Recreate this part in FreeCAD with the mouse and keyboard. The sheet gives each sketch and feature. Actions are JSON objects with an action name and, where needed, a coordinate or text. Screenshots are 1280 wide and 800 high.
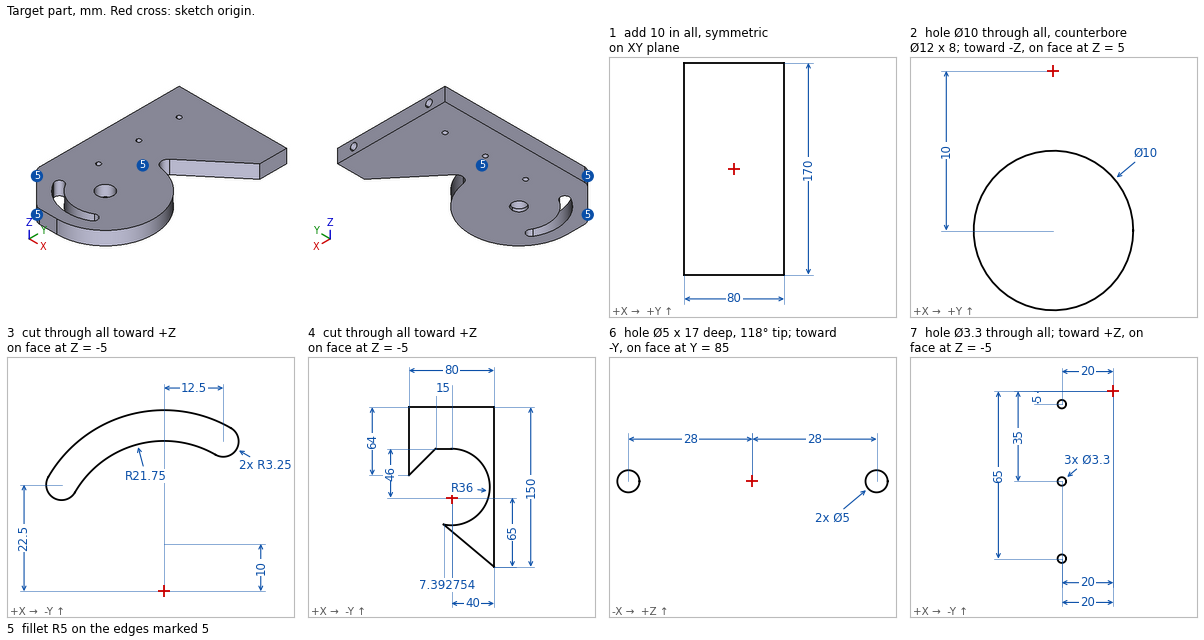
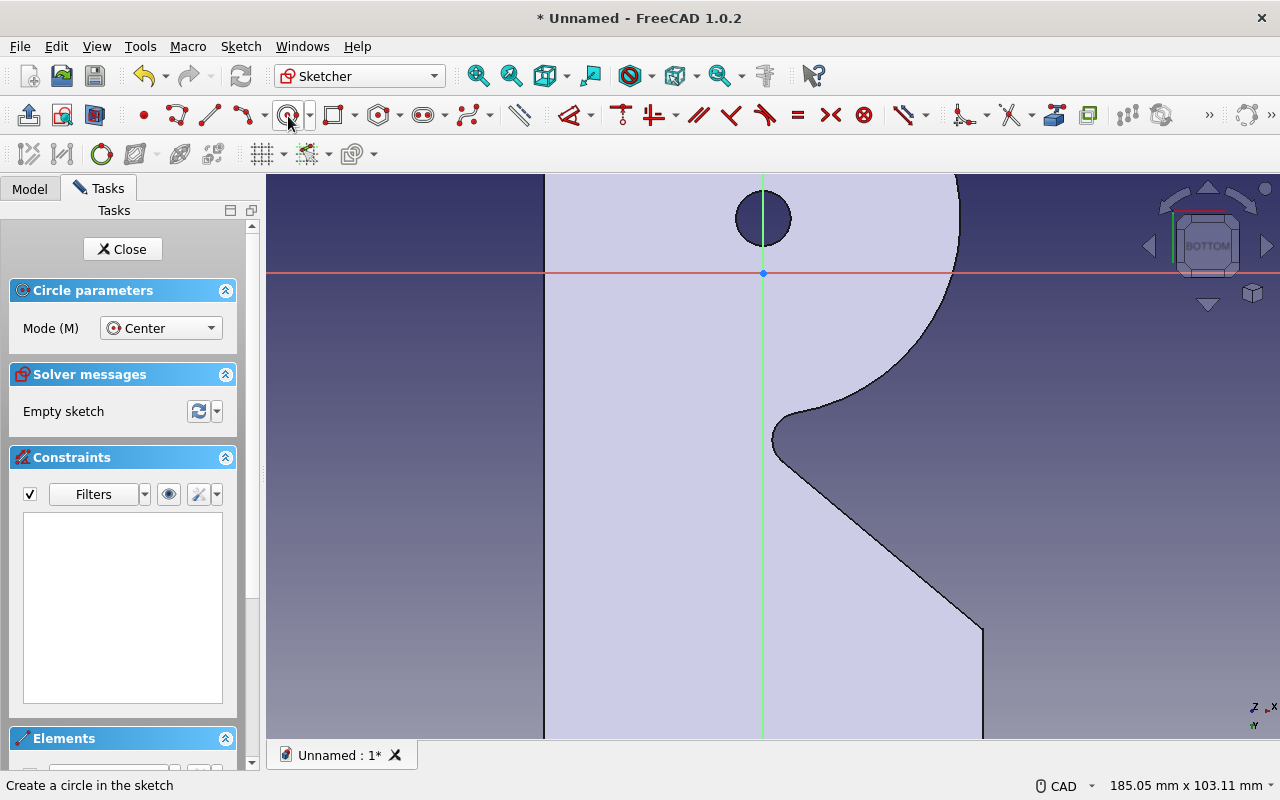
{"action": "scroll", "coordinate": [654, 465], "scroll_direction": "up", "scroll_amount": 5}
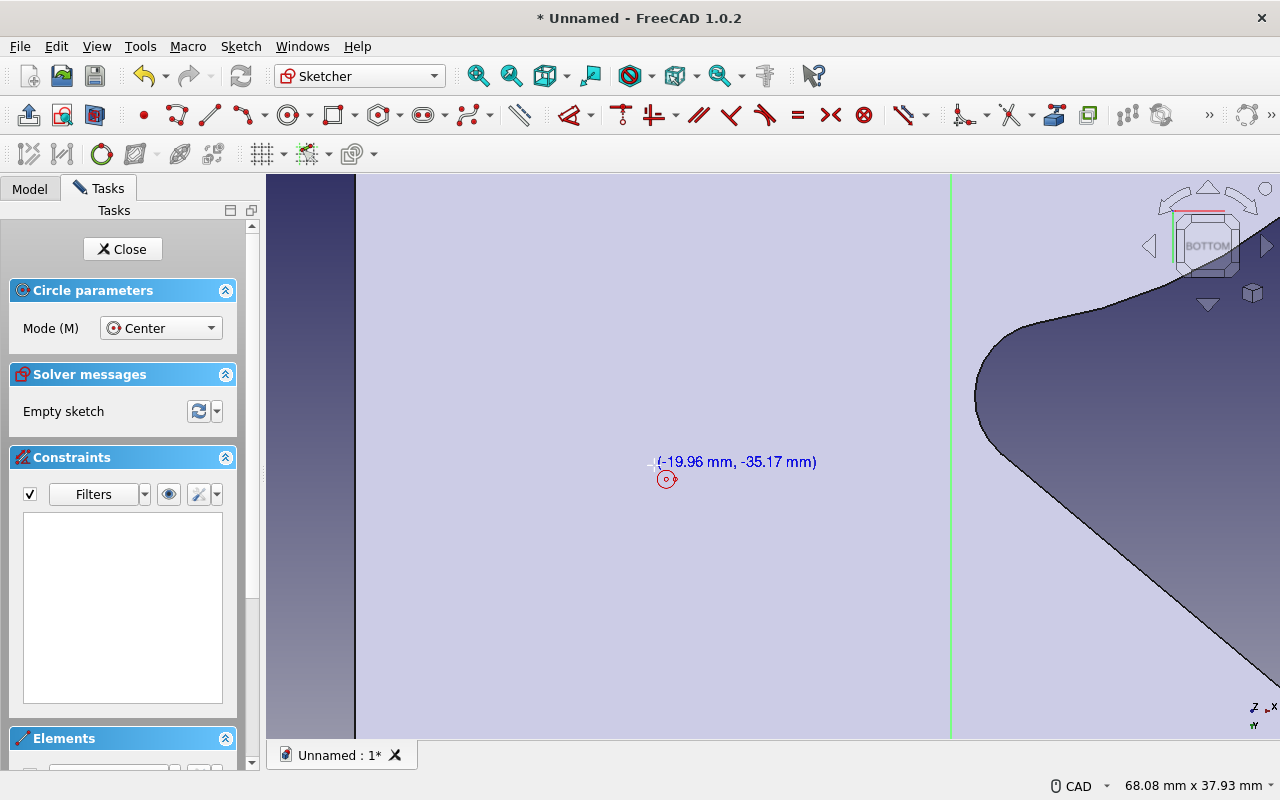
{"action": "left_click", "coordinate": [653, 464]}
{"action": "left_click", "coordinate": [670, 447]}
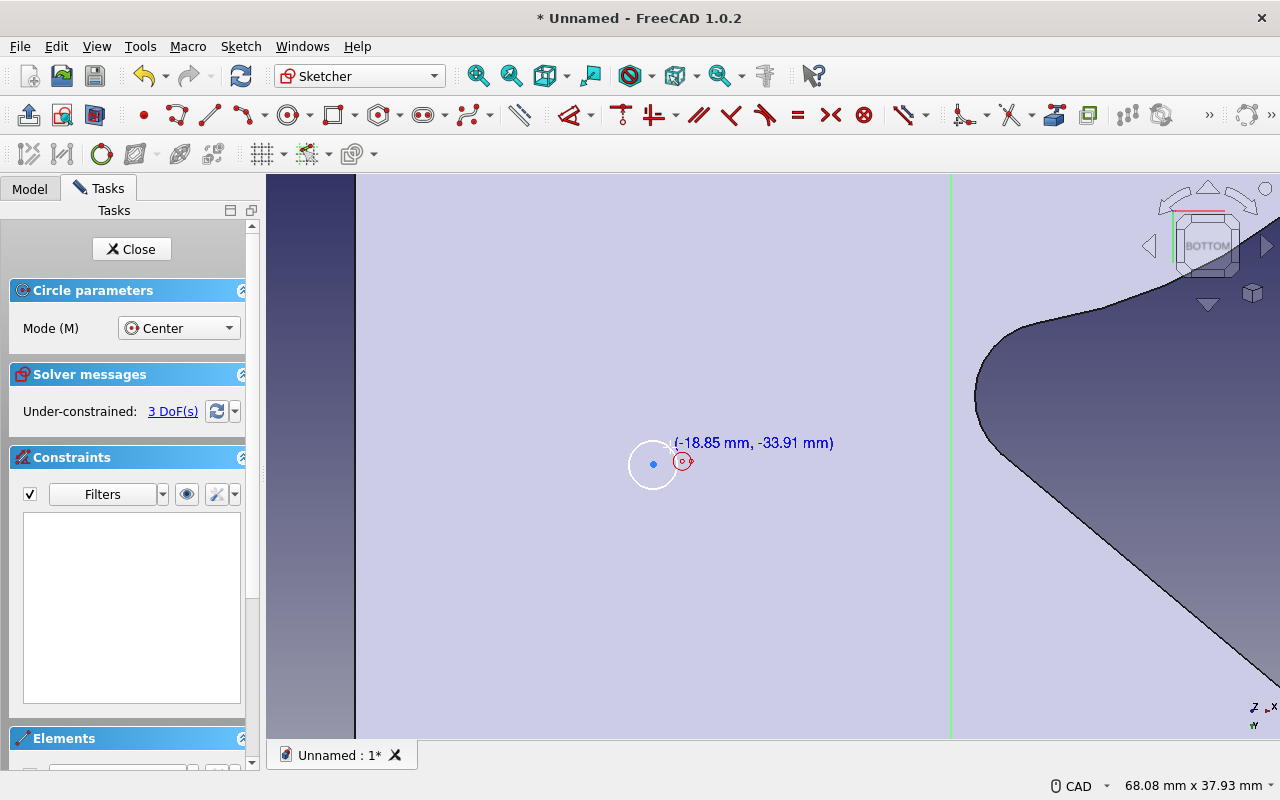
{"action": "scroll", "coordinate": [655, 466], "scroll_direction": "down", "scroll_amount": 5}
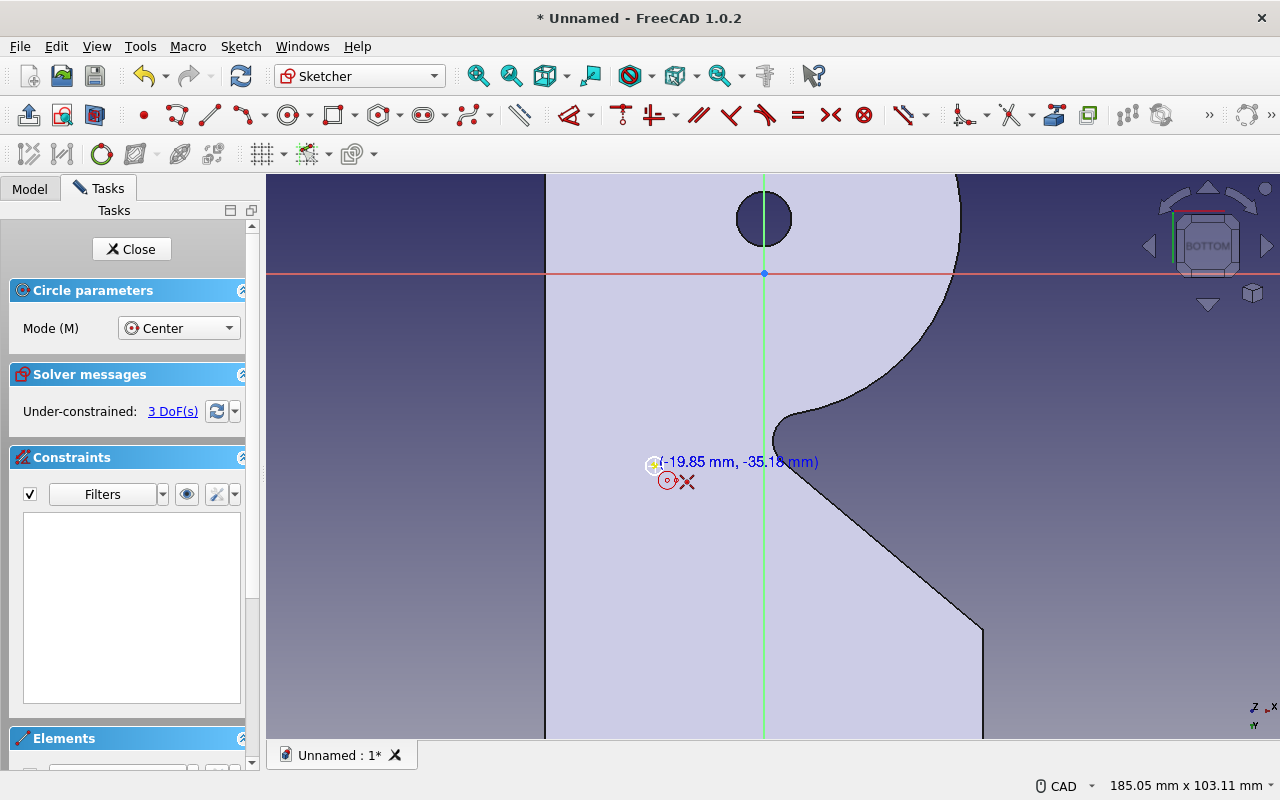
{"action": "scroll", "coordinate": [654, 630], "scroll_direction": "up", "scroll_amount": 5}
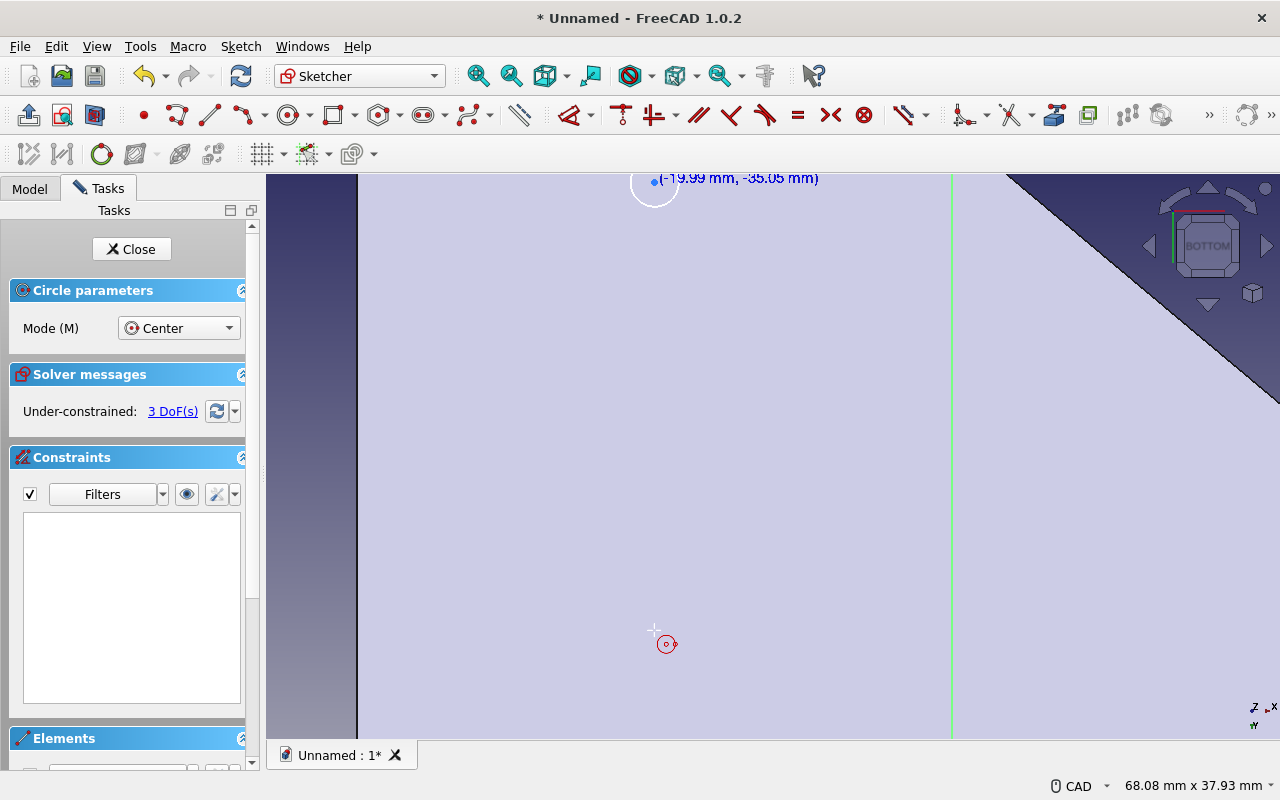
{"action": "left_click", "coordinate": [655, 629]}
{"action": "left_click", "coordinate": [672, 611]}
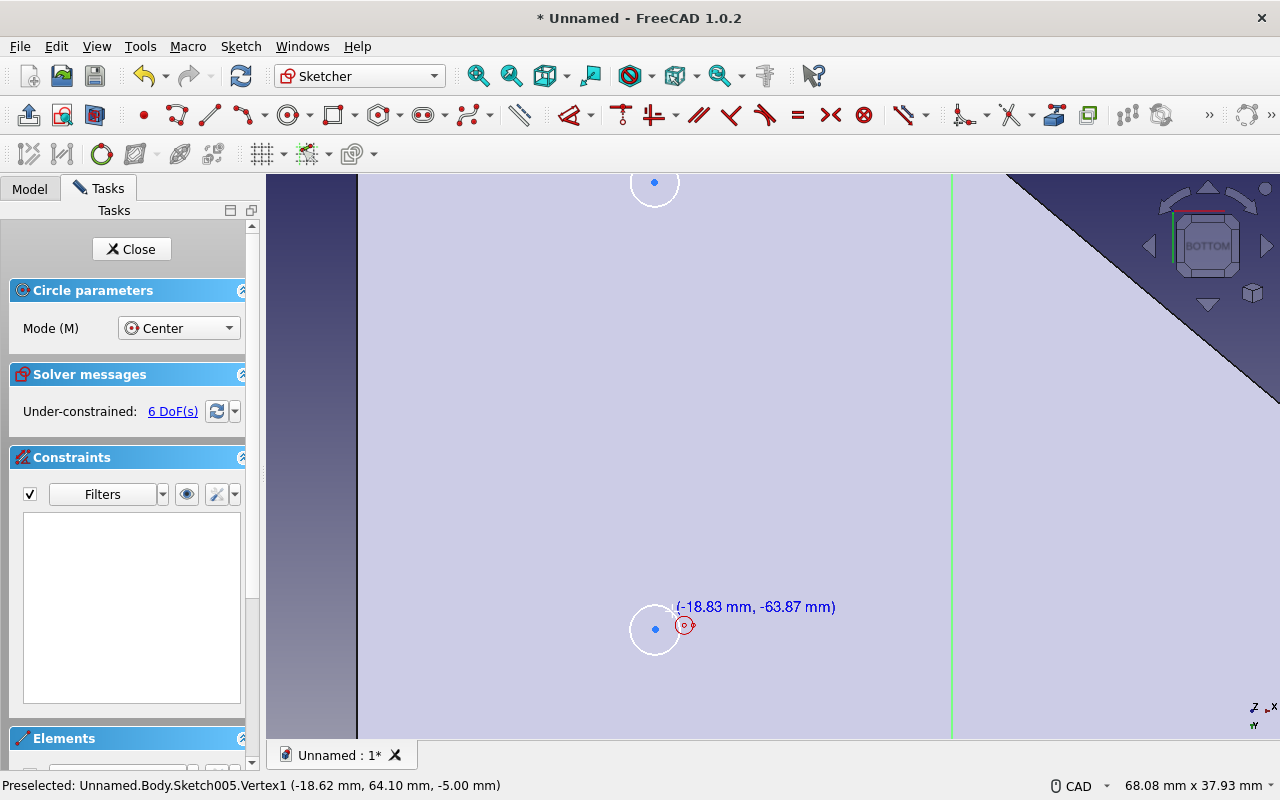
{"action": "scroll", "coordinate": [654, 631], "scroll_direction": "down", "scroll_amount": 5}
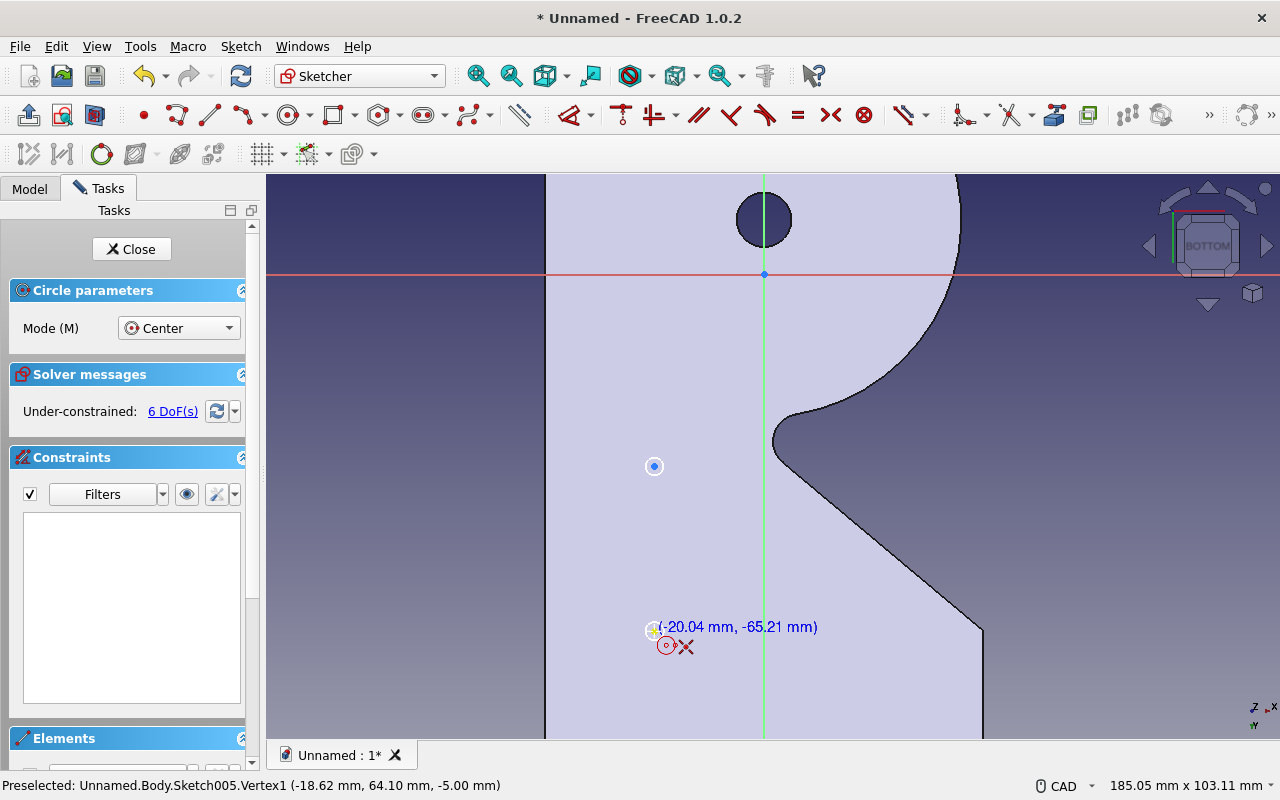
{"action": "scroll", "coordinate": [654, 302], "scroll_direction": "up", "scroll_amount": 5}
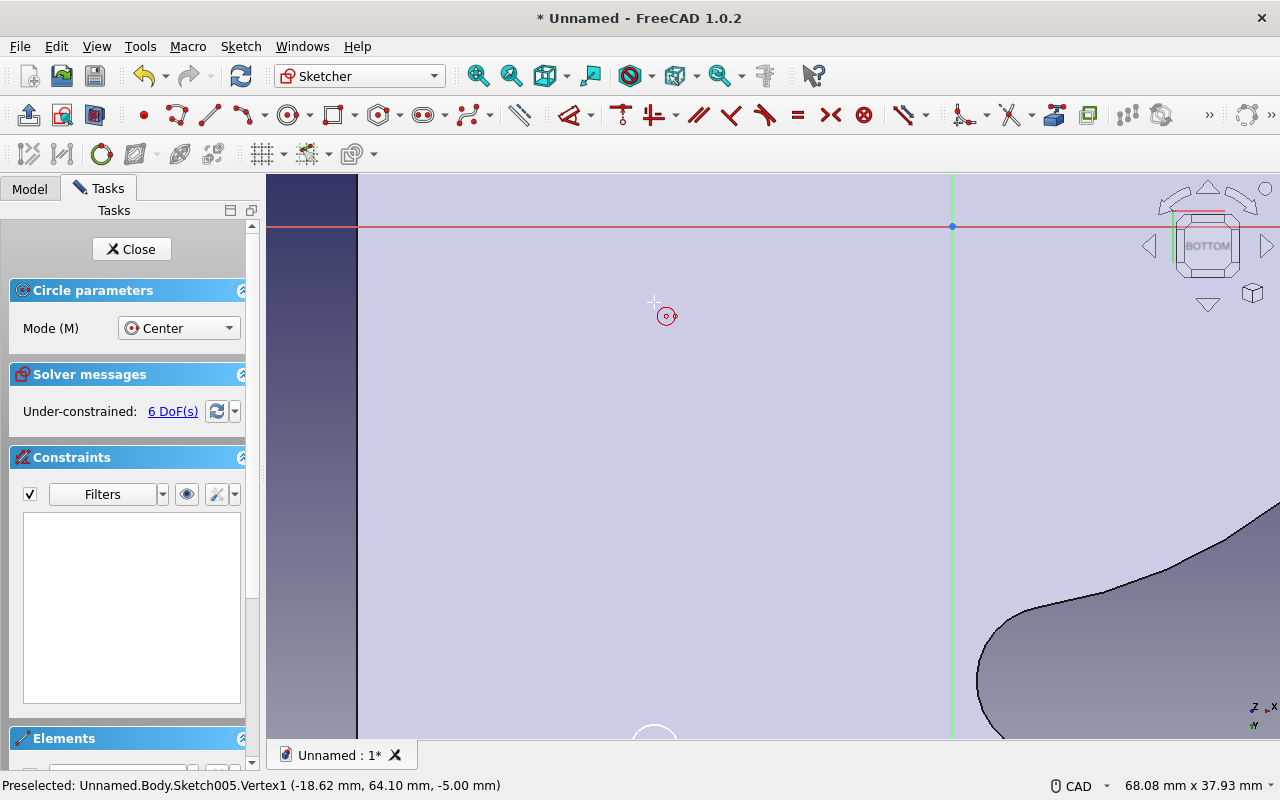
{"action": "left_click", "coordinate": [655, 301]}
{"action": "left_click", "coordinate": [672, 284]}
{"action": "key", "text": "Escape"}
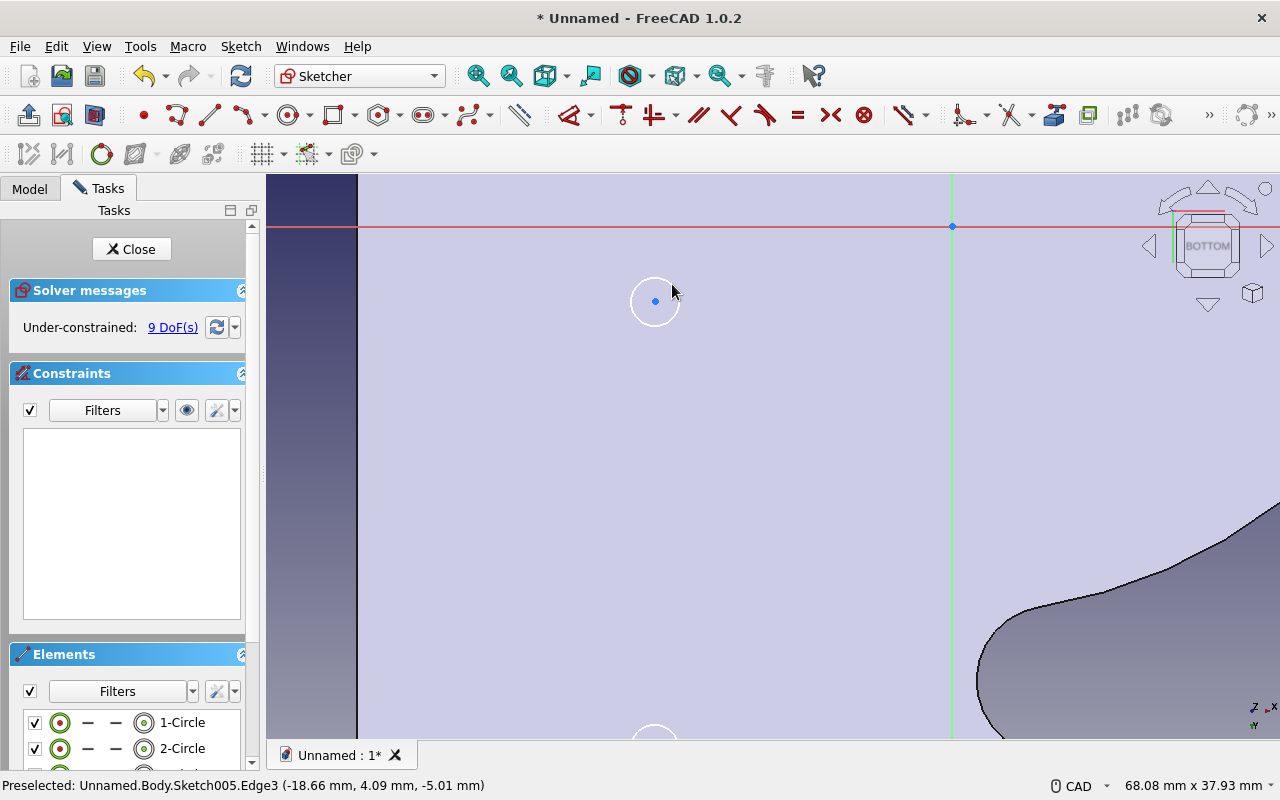
{"action": "scroll", "coordinate": [654, 301], "scroll_direction": "down", "scroll_amount": 5}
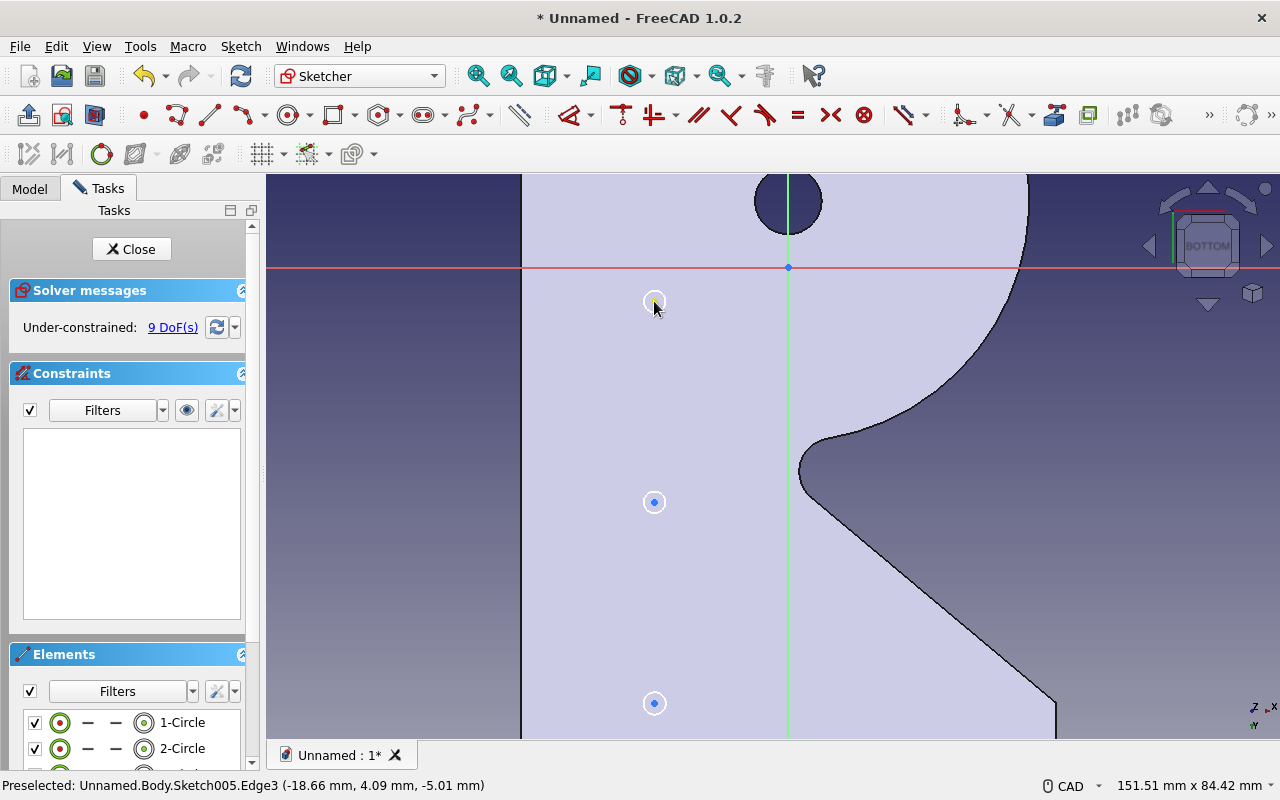
{"action": "scroll", "coordinate": [661, 460], "scroll_direction": "up", "scroll_amount": 3}